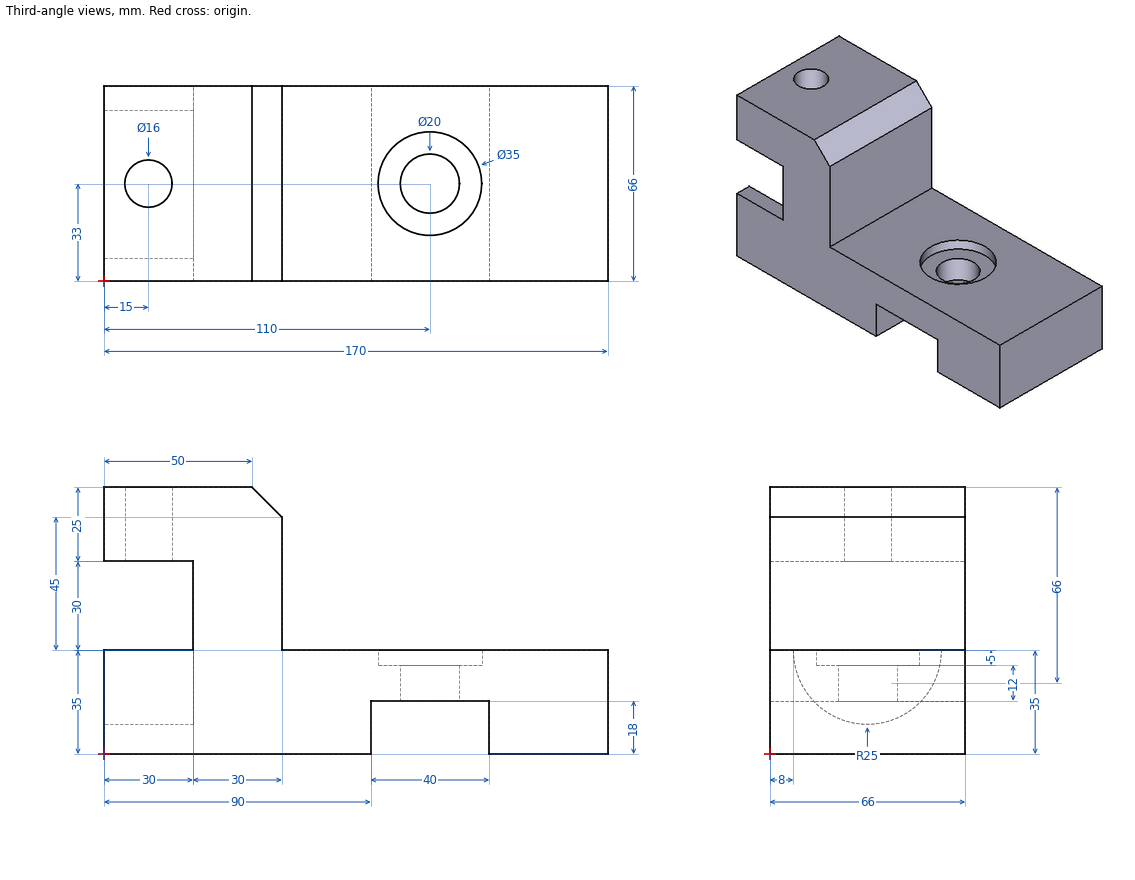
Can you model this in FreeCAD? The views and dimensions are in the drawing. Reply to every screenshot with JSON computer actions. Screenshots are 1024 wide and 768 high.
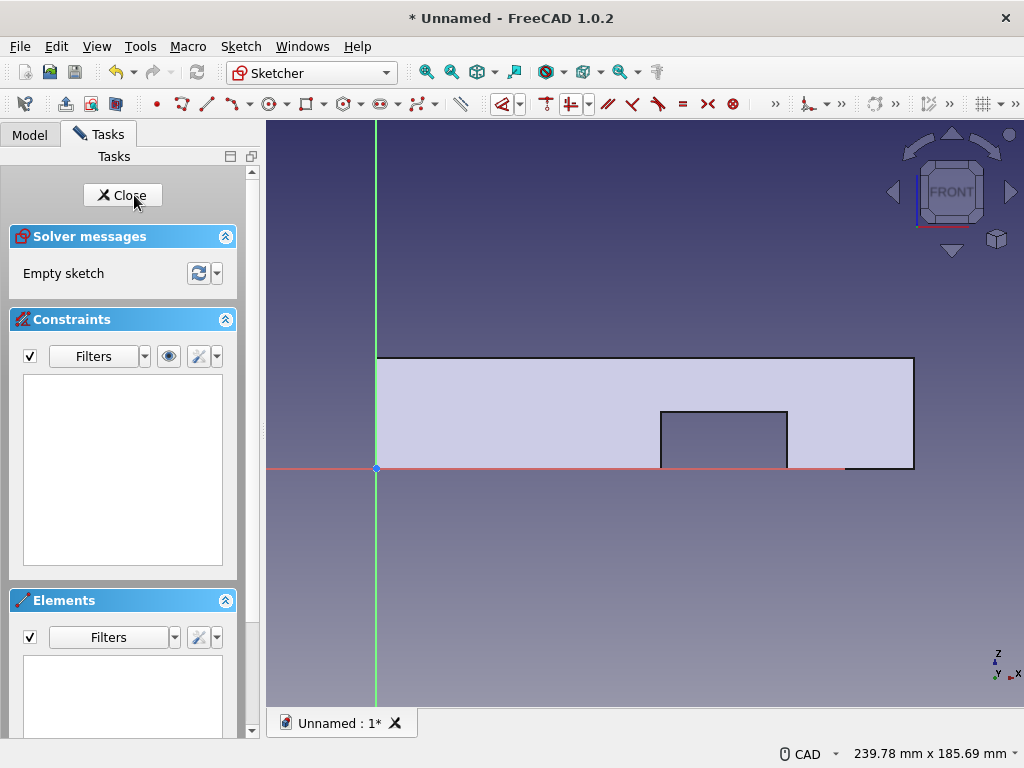
{"action": "left_click", "coordinate": [471, 358]}
{"action": "left_click", "coordinate": [566, 358]}
{"action": "left_click", "coordinate": [566, 216]}
{"action": "left_click", "coordinate": [534, 184]}
{"action": "left_click", "coordinate": [376, 184]}
{"action": "left_click", "coordinate": [385, 263]}
{"action": "left_click", "coordinate": [471, 263]}
{"action": "left_click", "coordinate": [471, 359]}
{"action": "key", "text": "Escape"}
{"action": "key", "text": "Escape"}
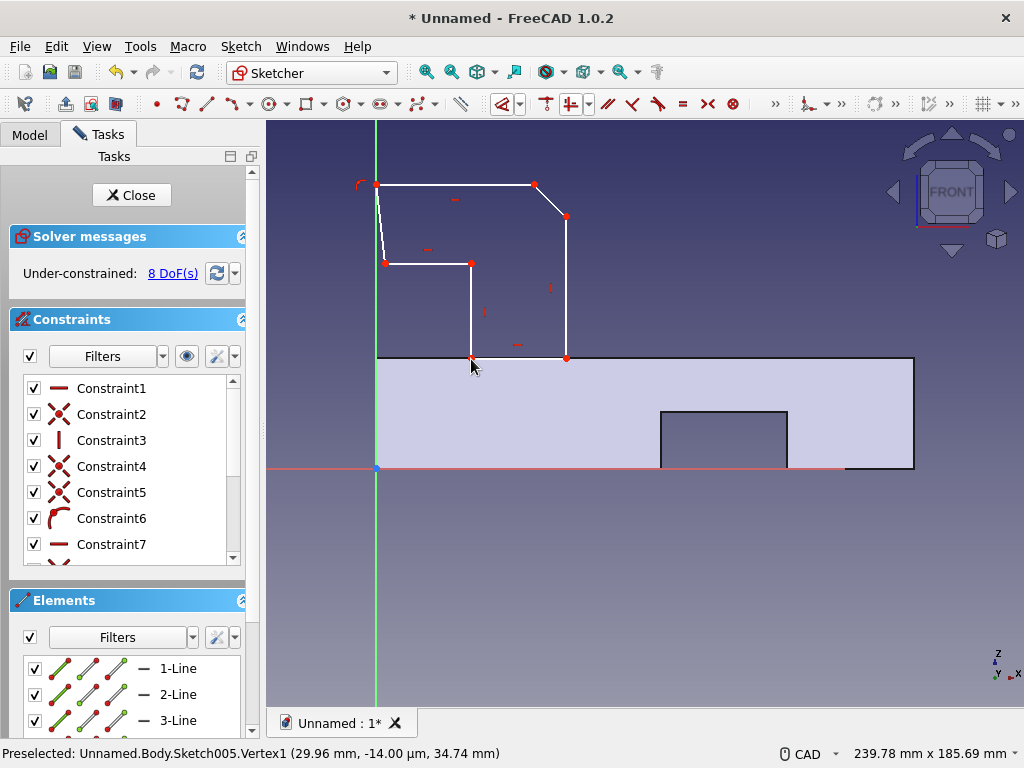
{"action": "left_click", "coordinate": [379, 209]}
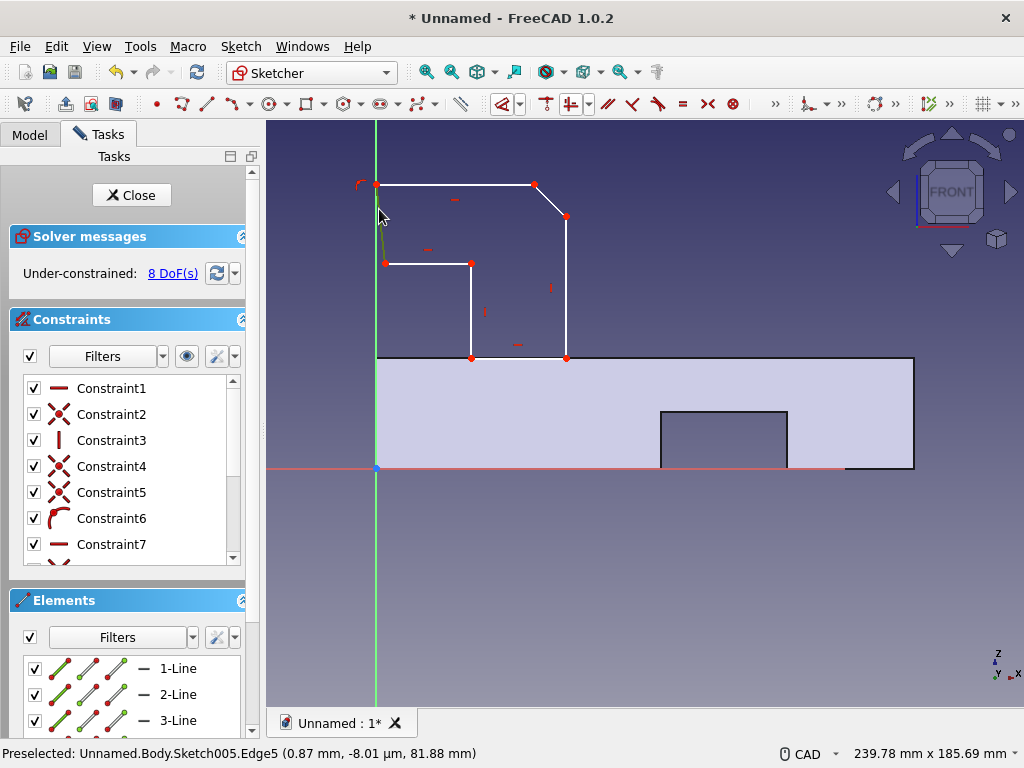
{"action": "key", "text": "v"}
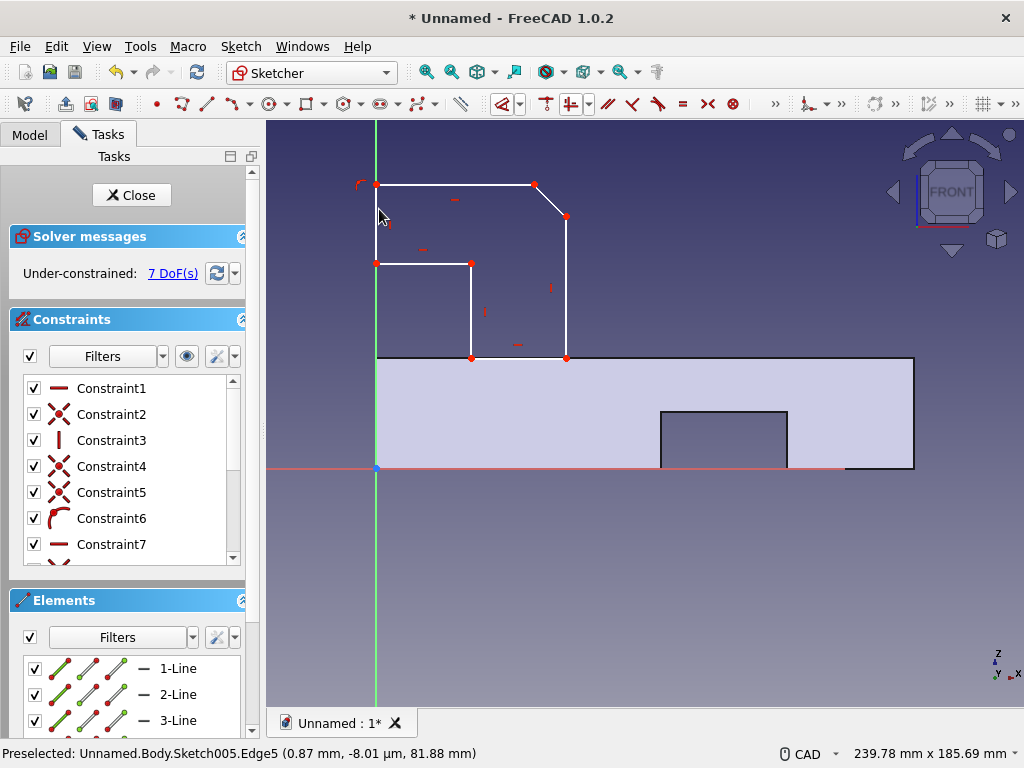
{"action": "left_click", "coordinate": [499, 359]}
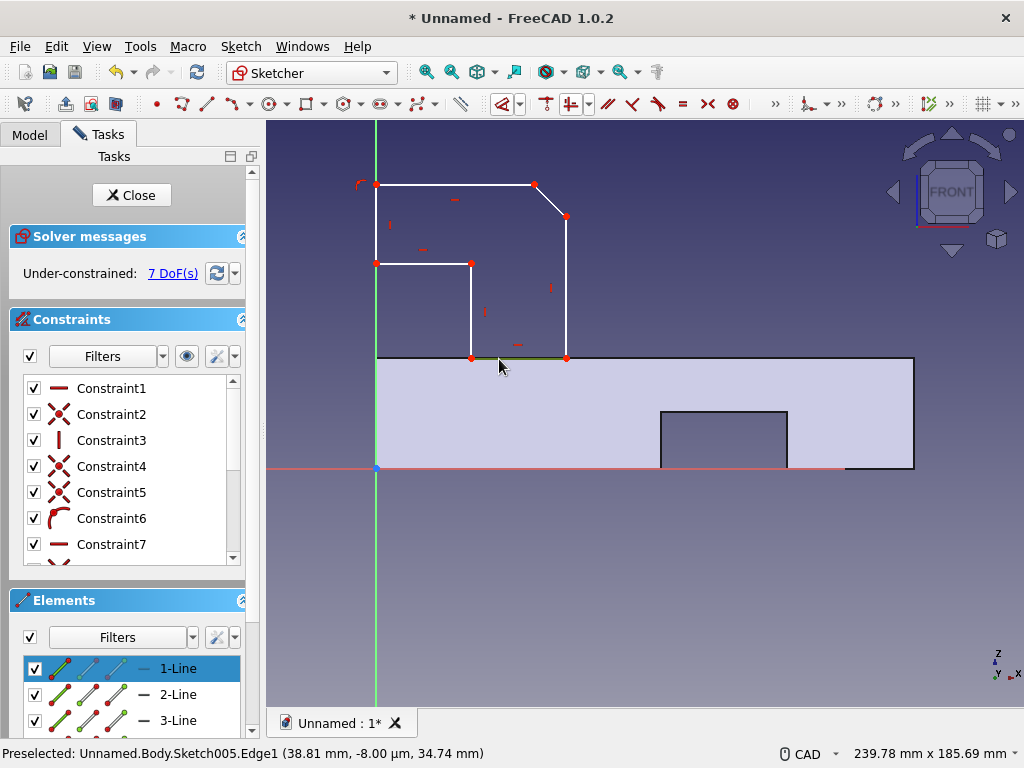
{"action": "left_click", "coordinate": [520, 104]}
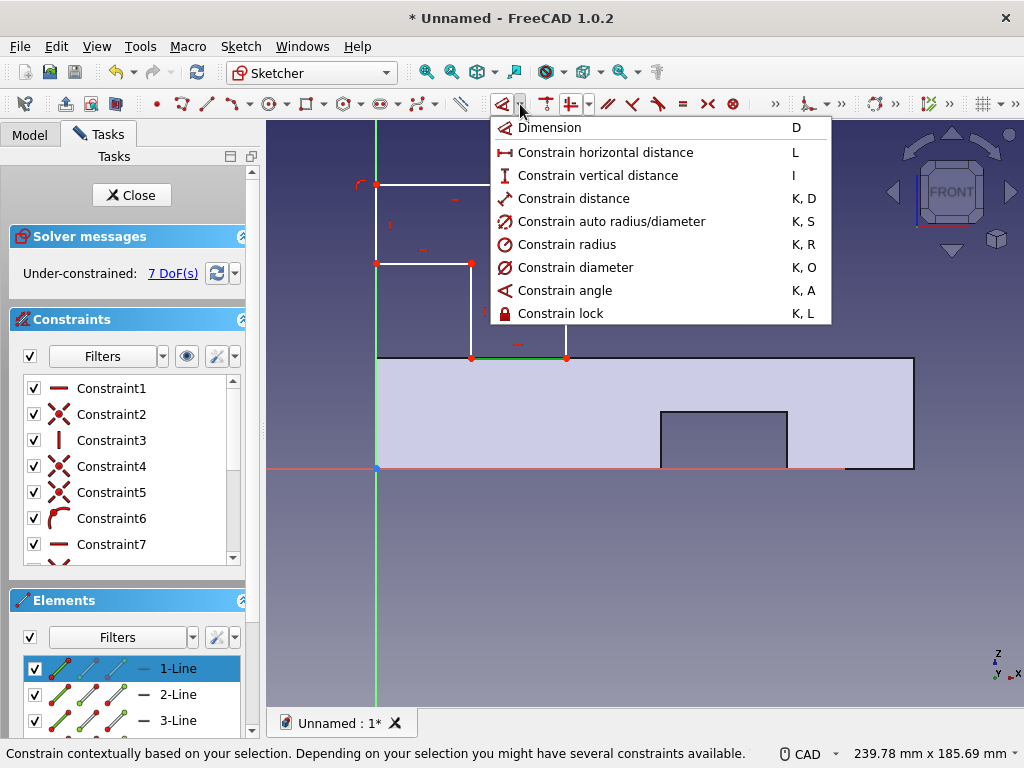
{"action": "left_click", "coordinate": [661, 152]}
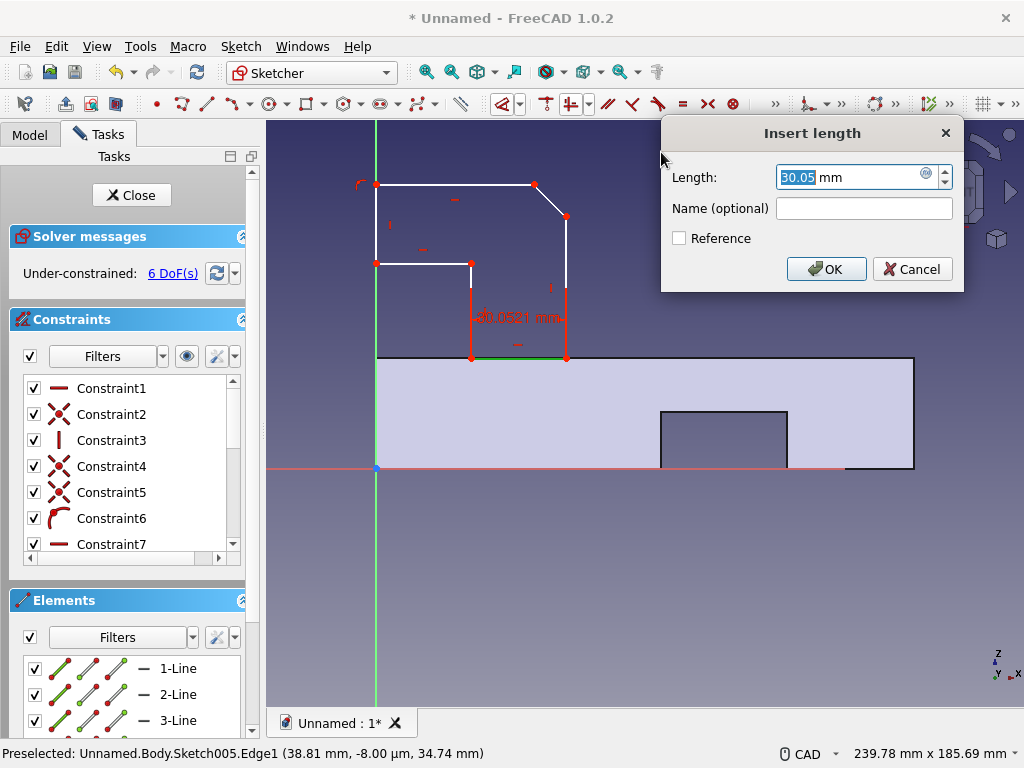
{"action": "type", "text": "30"}
{"action": "key", "text": "Return"}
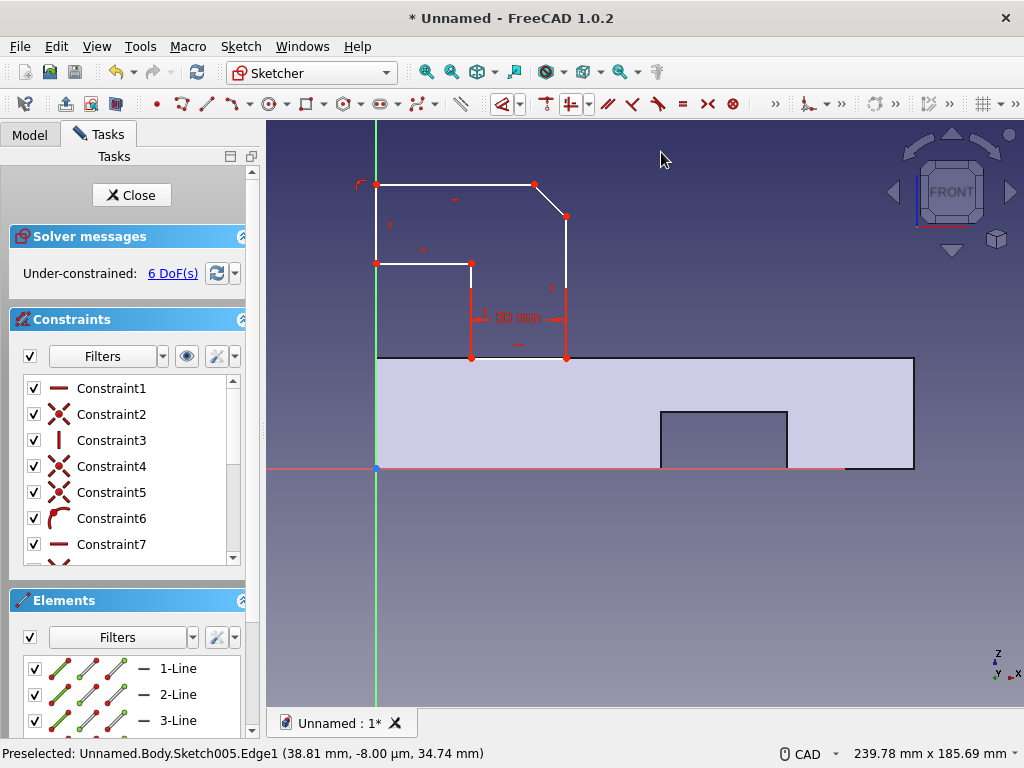
{"action": "left_click", "coordinate": [566, 316]}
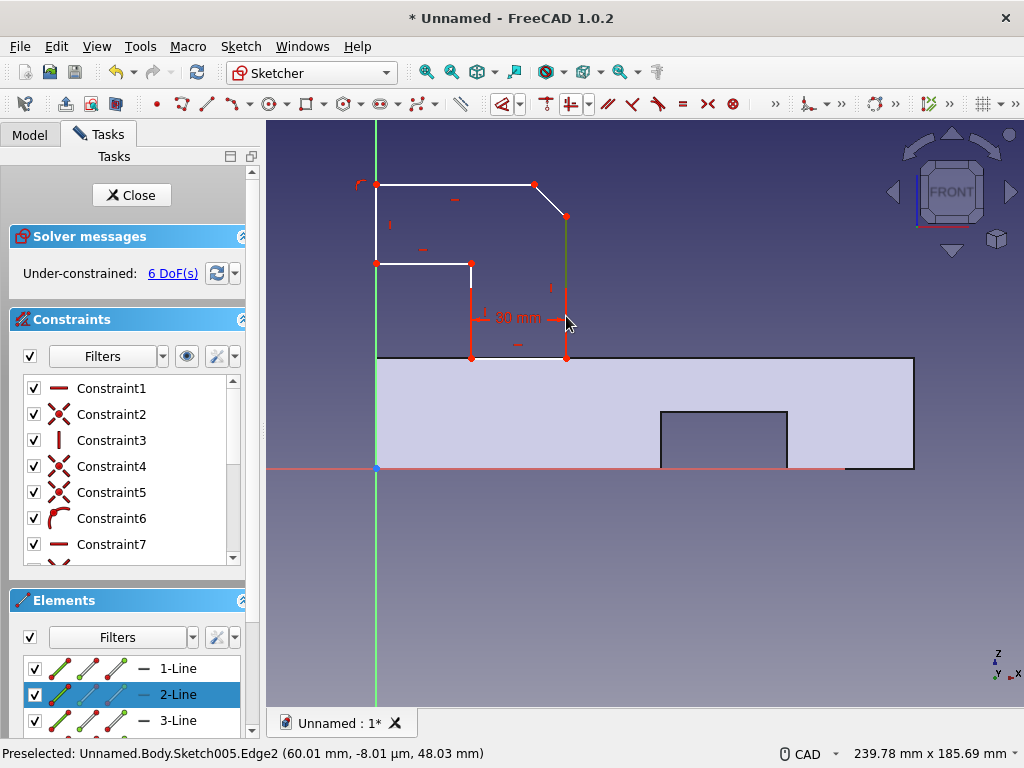
{"action": "key", "text": "i"}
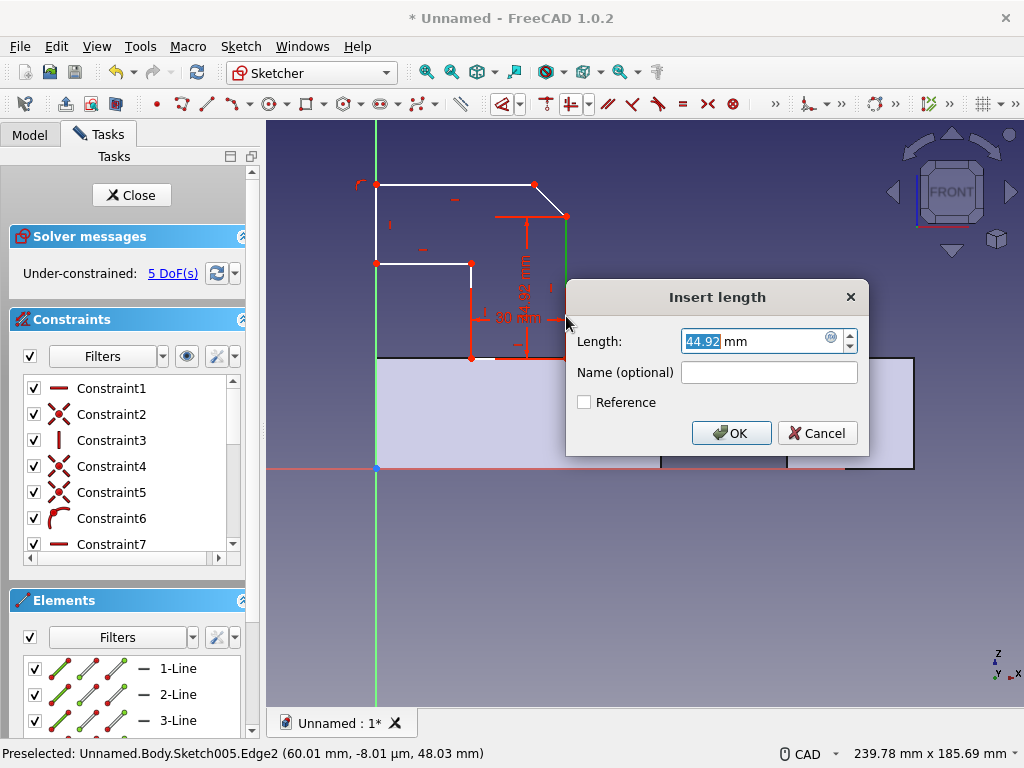
{"action": "type", "text": "45"}
{"action": "key", "text": "Return"}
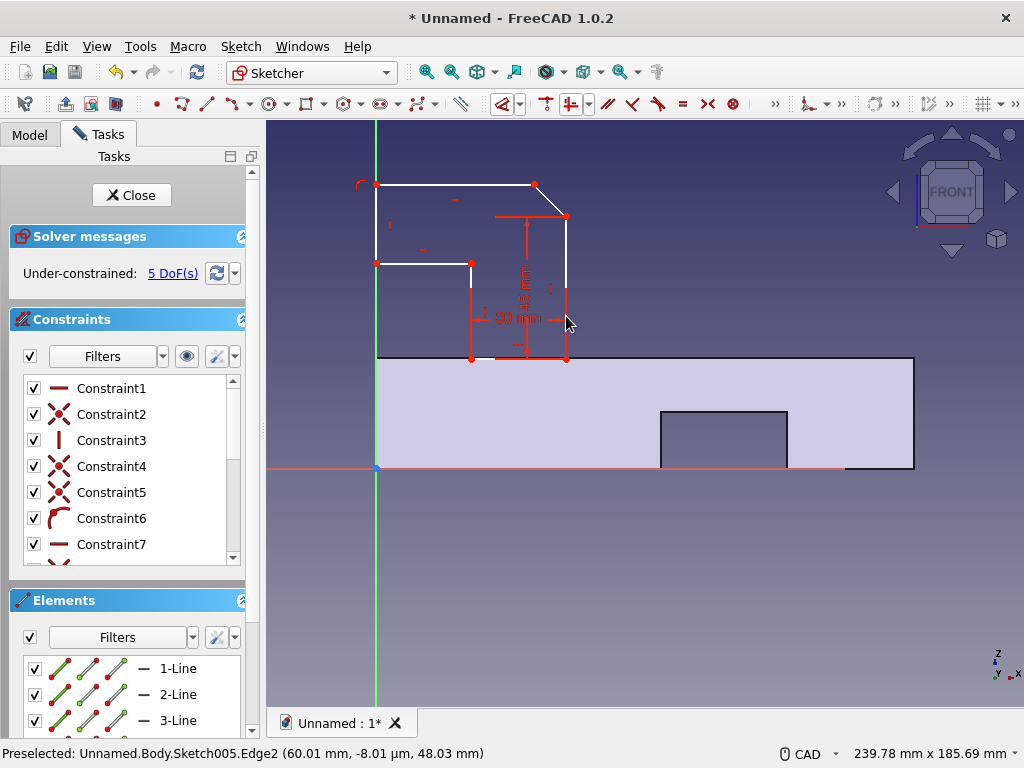
{"action": "left_click", "coordinate": [487, 185]}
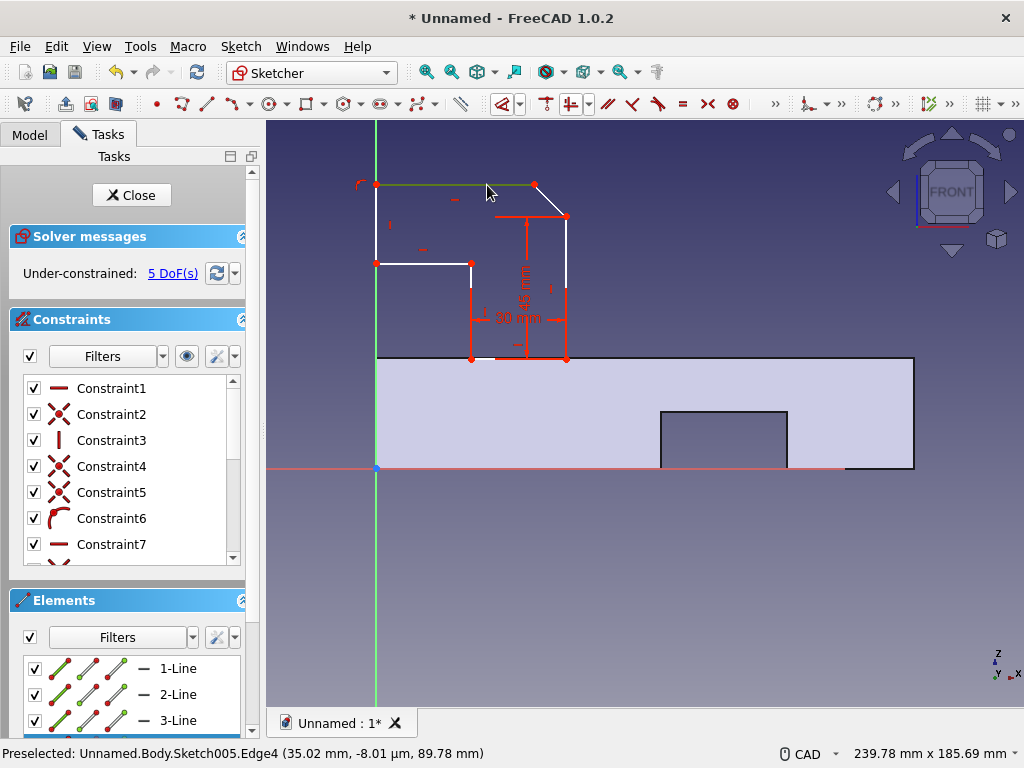
{"action": "key", "text": "l"}